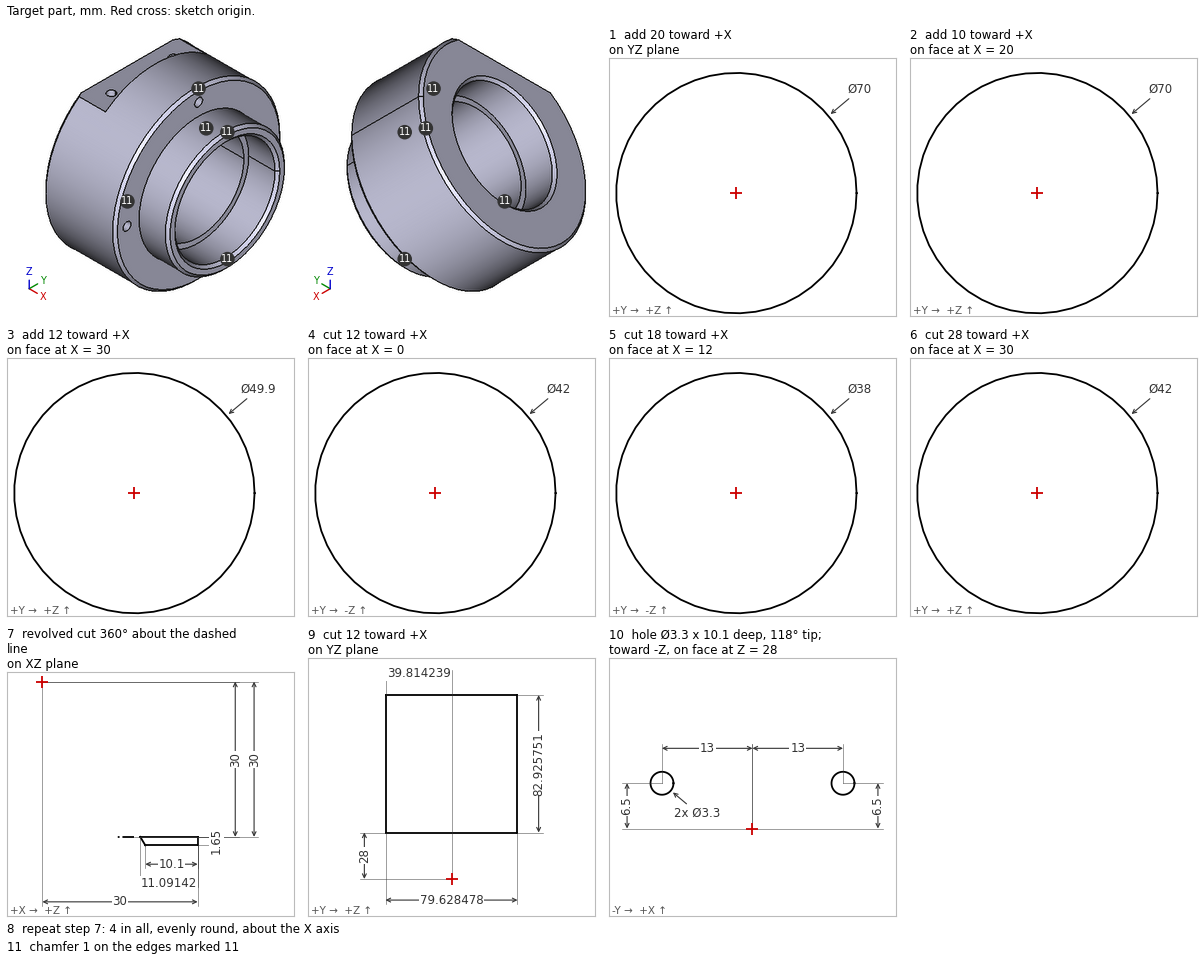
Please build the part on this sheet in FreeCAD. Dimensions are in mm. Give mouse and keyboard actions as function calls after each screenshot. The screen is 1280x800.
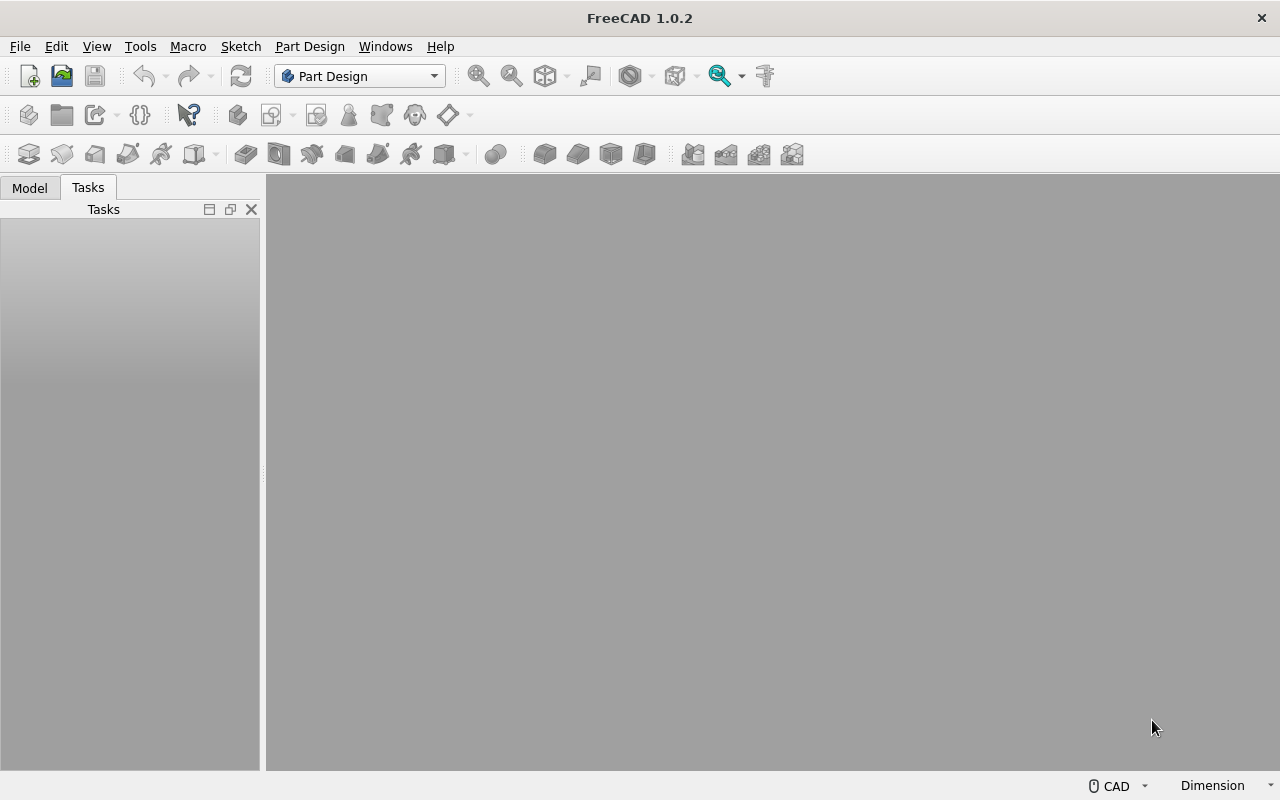
click(29, 76)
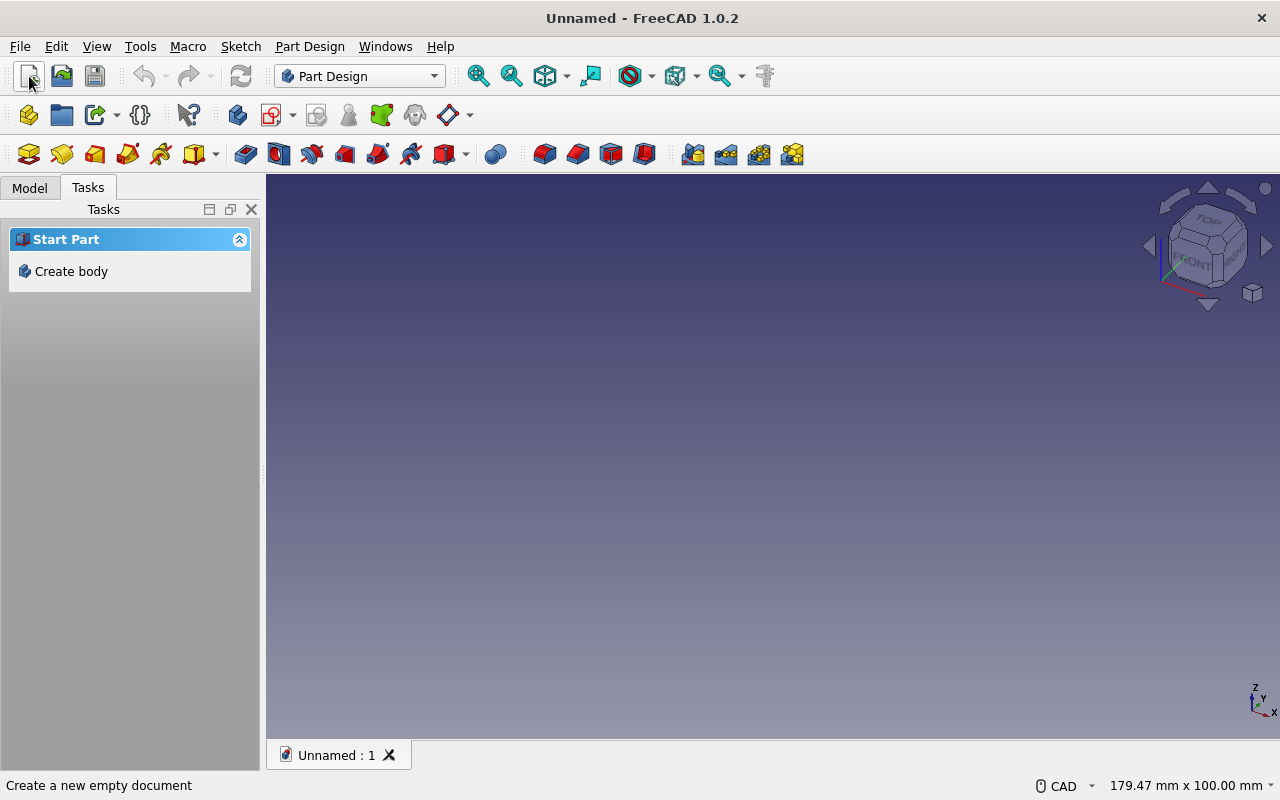
click(270, 116)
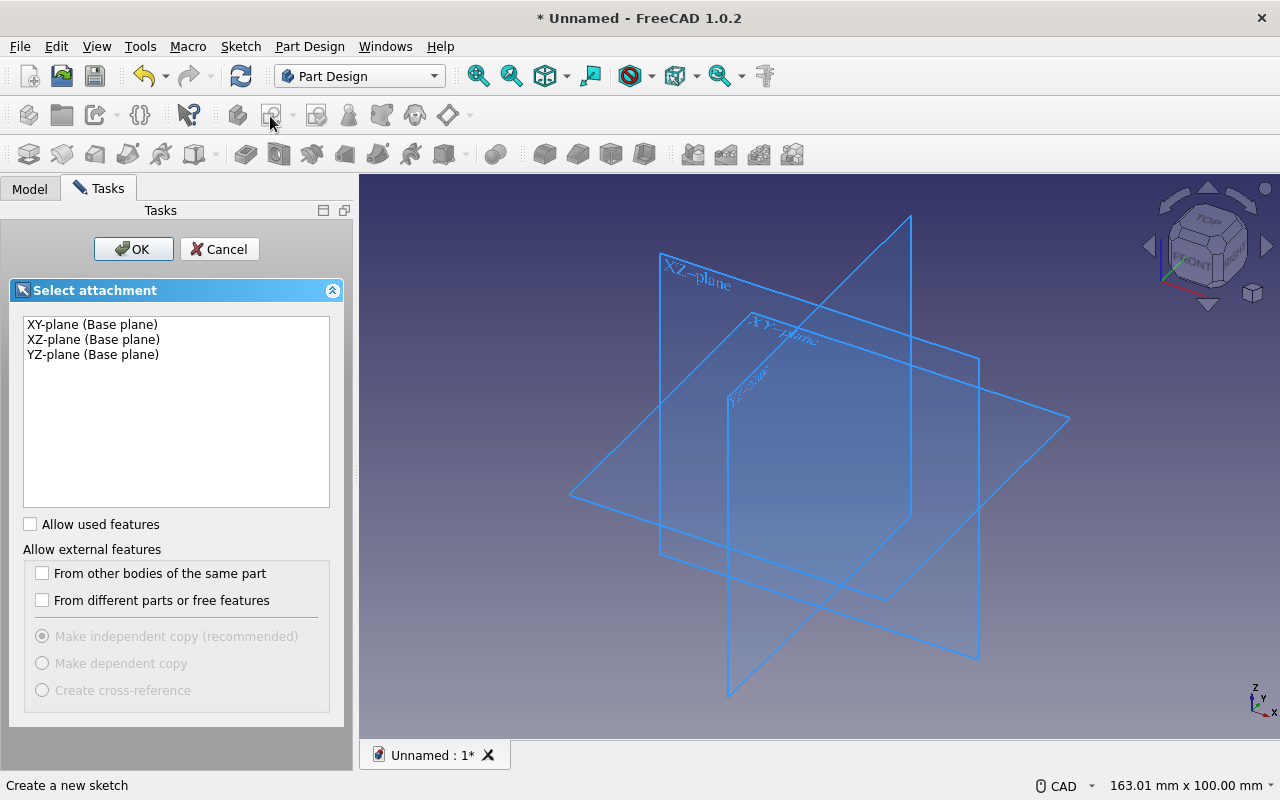
click(84, 354)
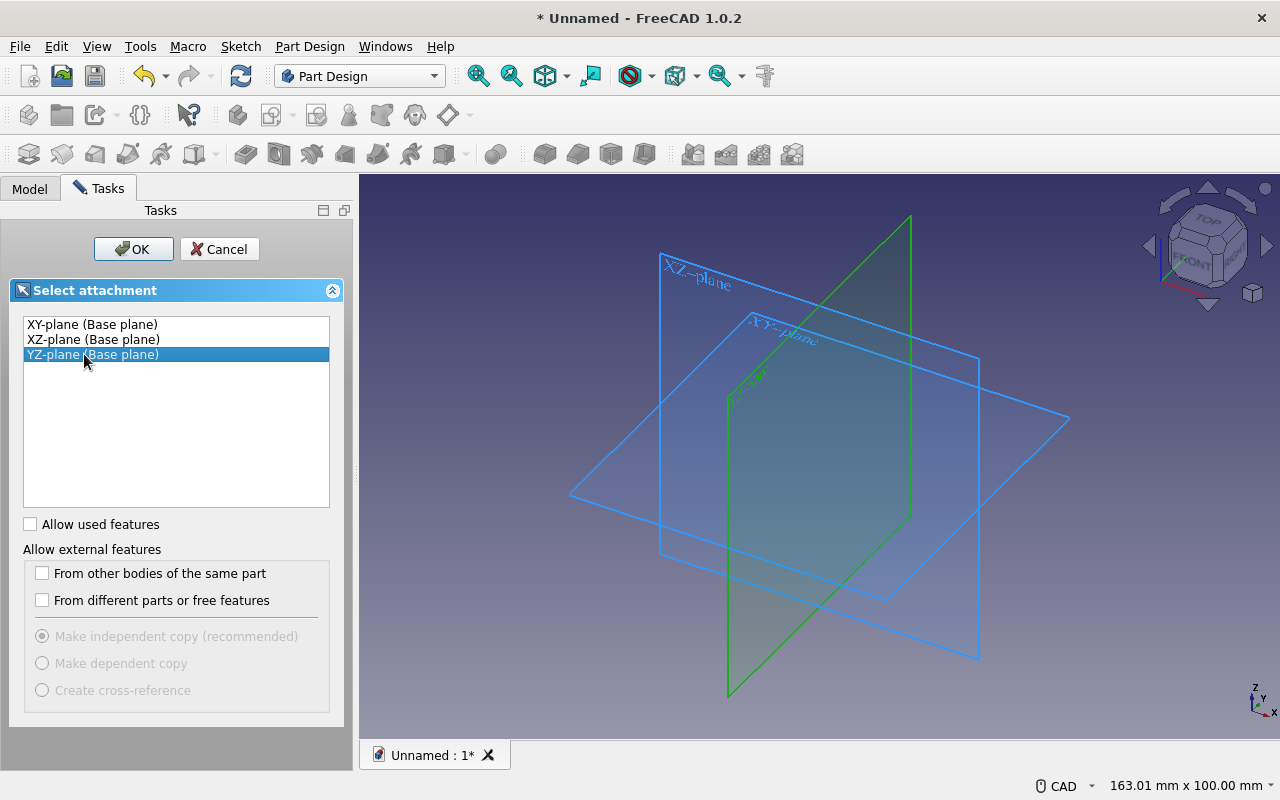
click(134, 249)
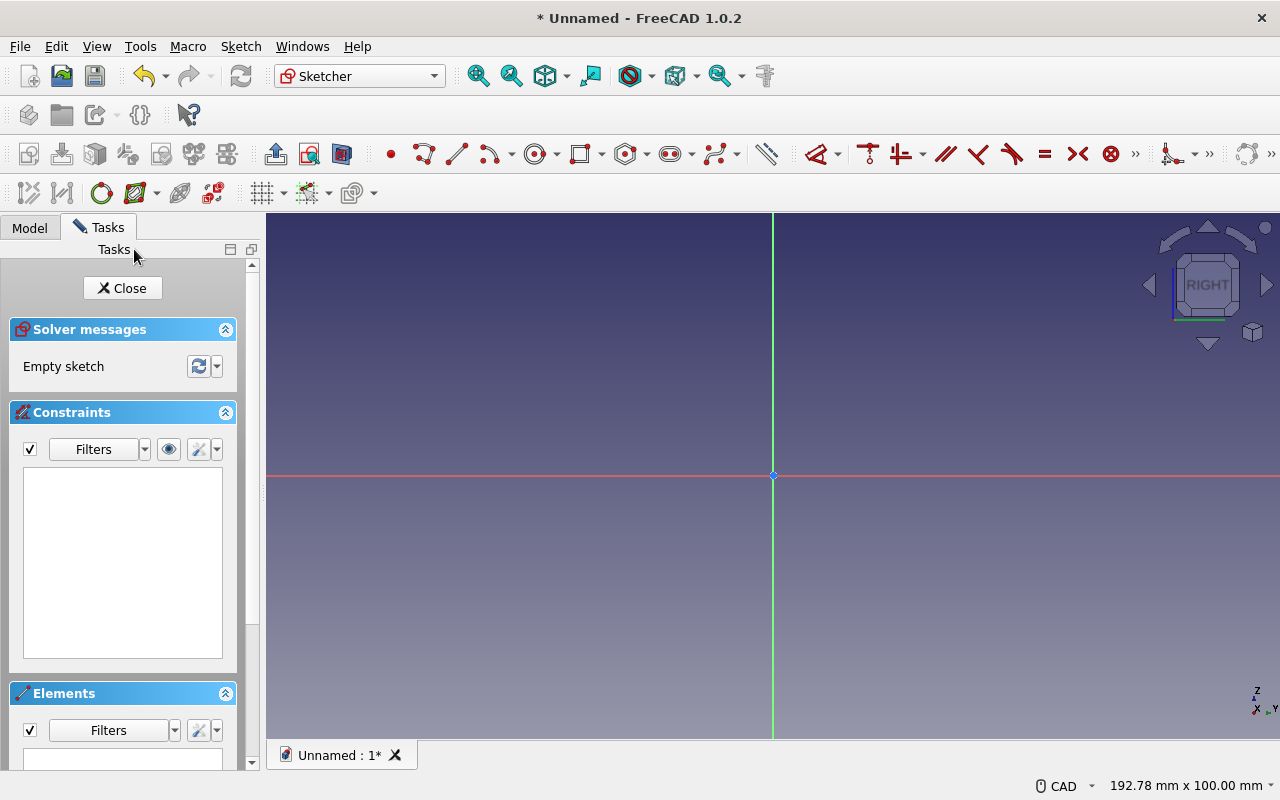
click(534, 154)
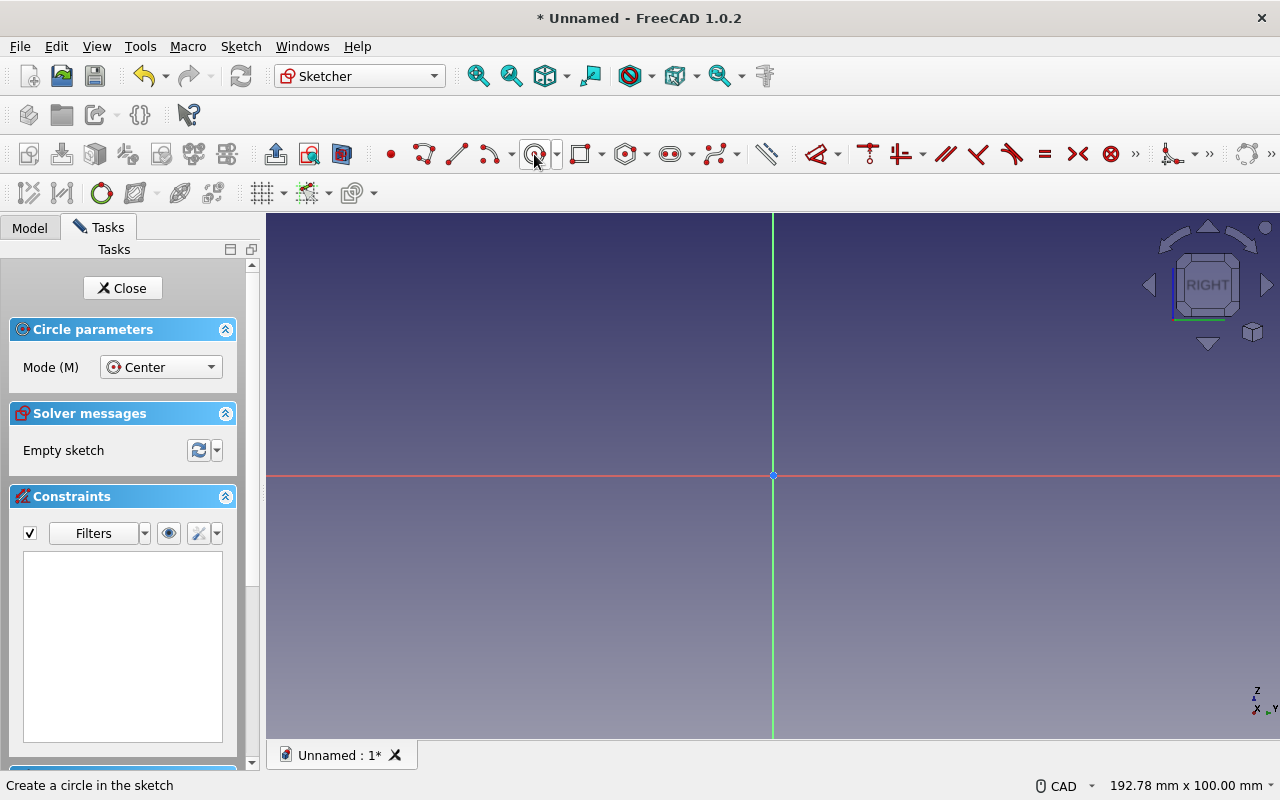
click(773, 476)
move(903, 346)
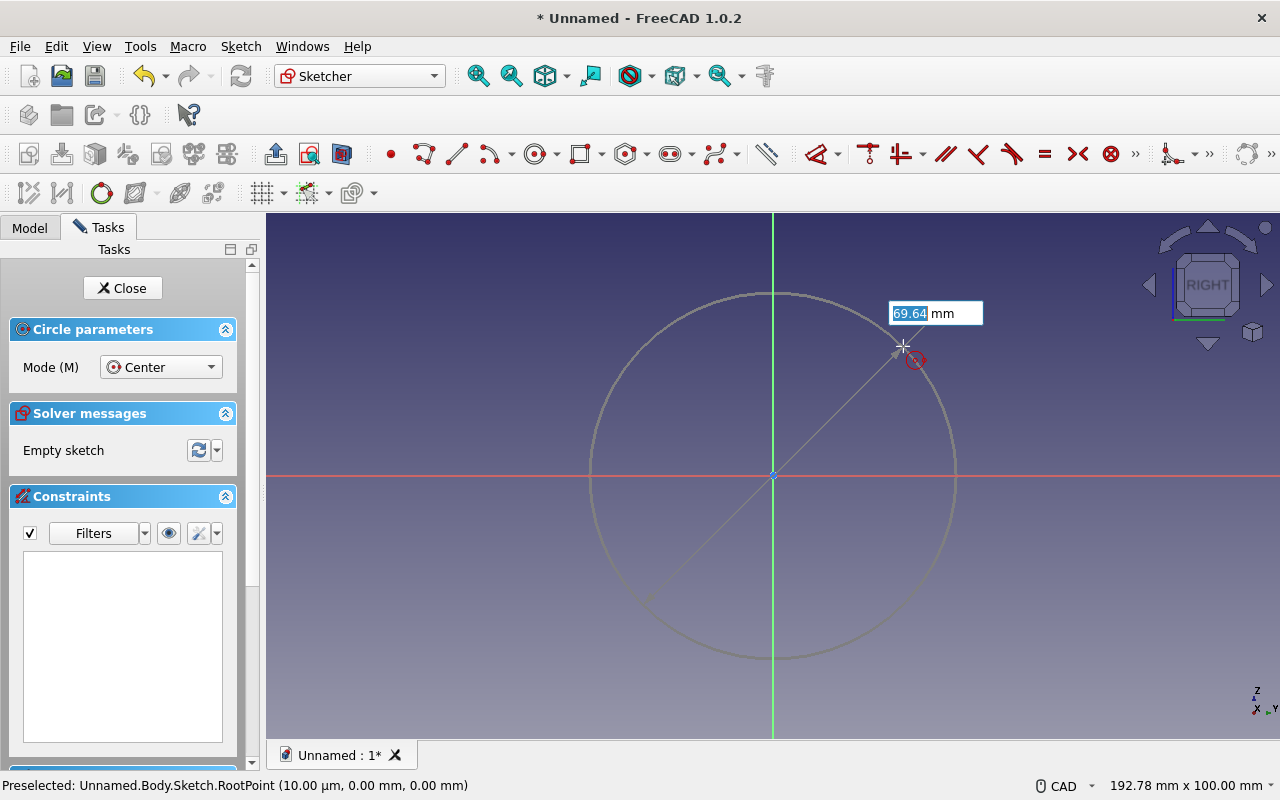
text(70)
key(Return)
key(Escape)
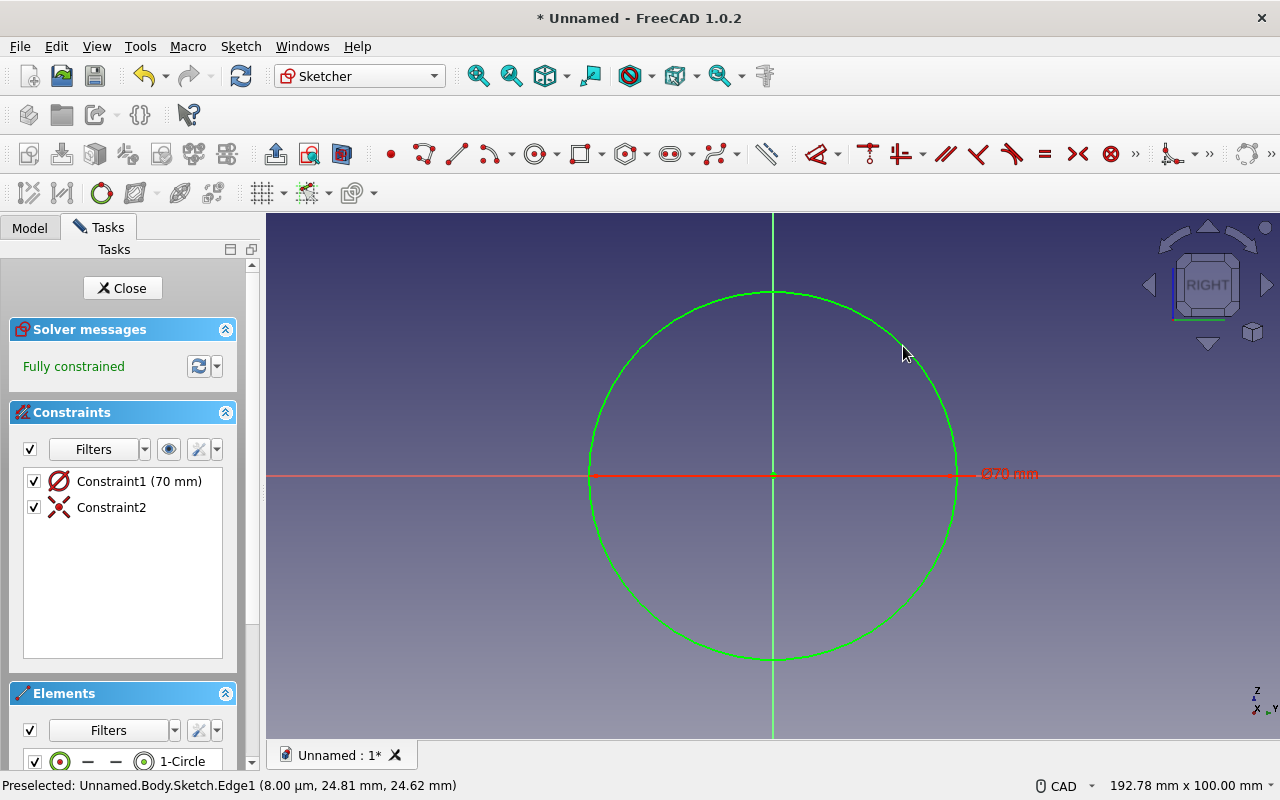
click(123, 288)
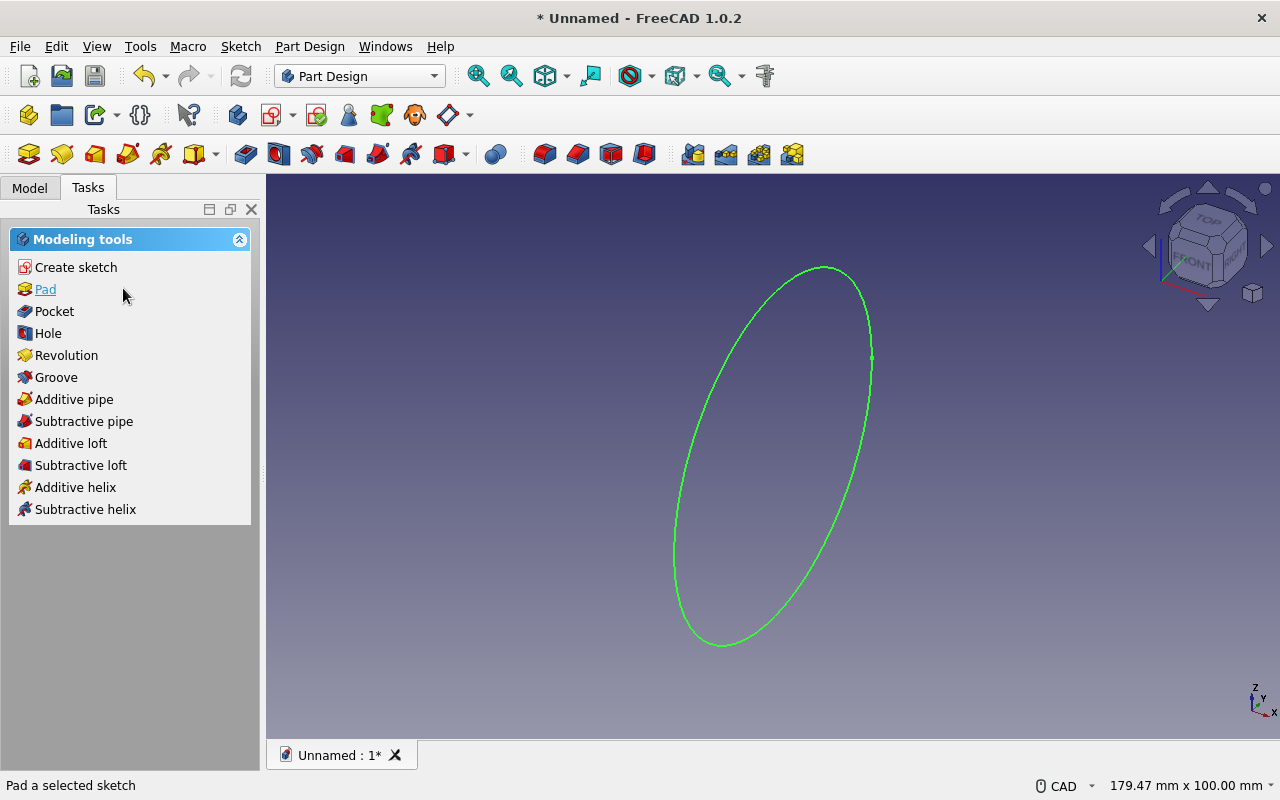
click(29, 154)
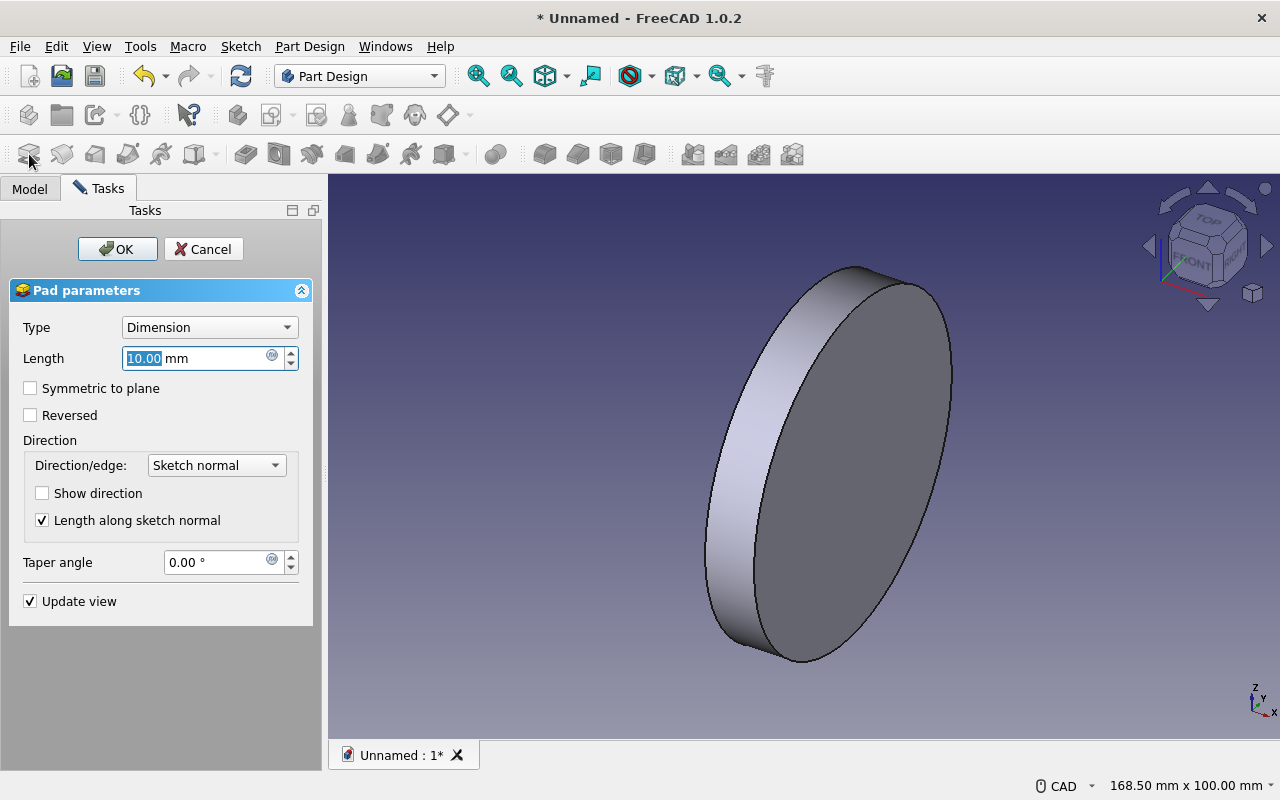
text(20)
key(Tab)